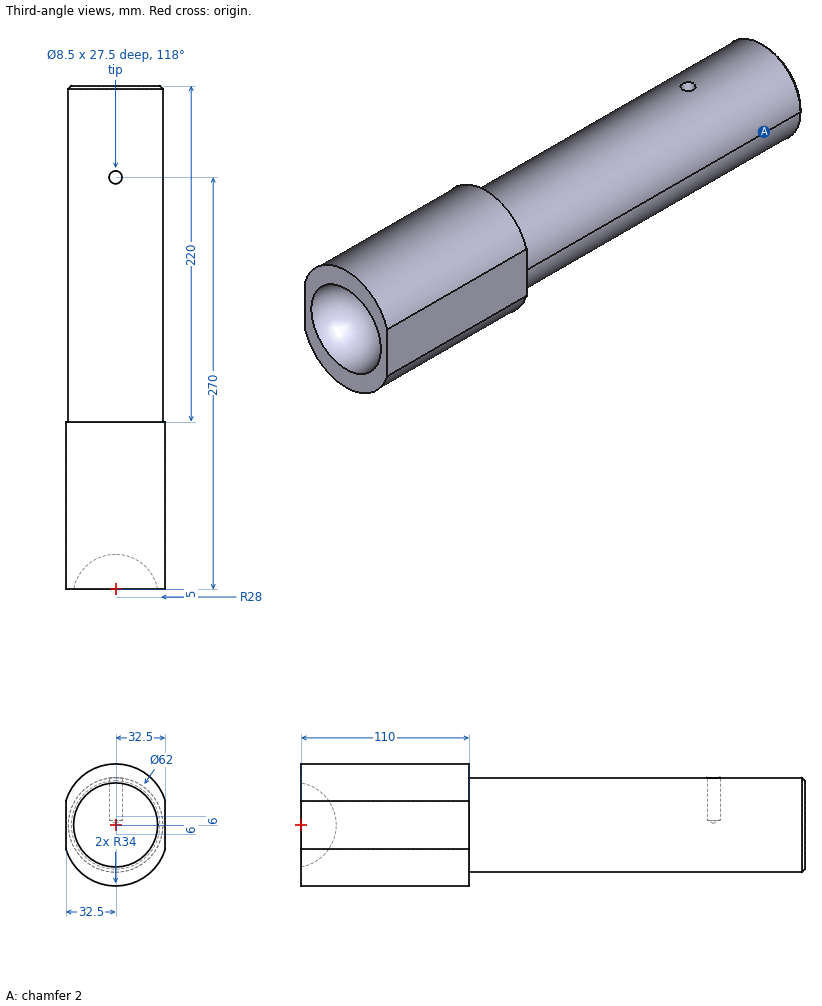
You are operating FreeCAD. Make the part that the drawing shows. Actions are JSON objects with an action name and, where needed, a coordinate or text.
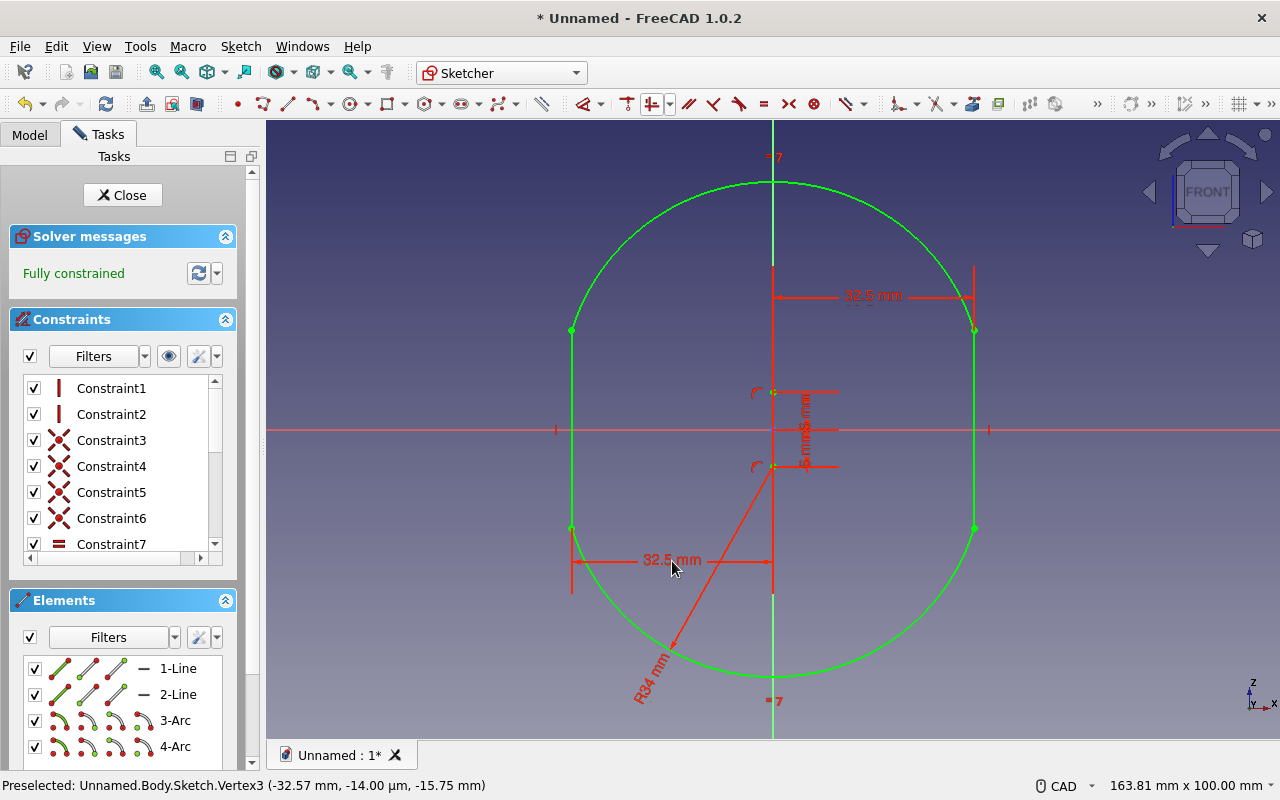
{"action": "left_click", "coordinate": [123, 195]}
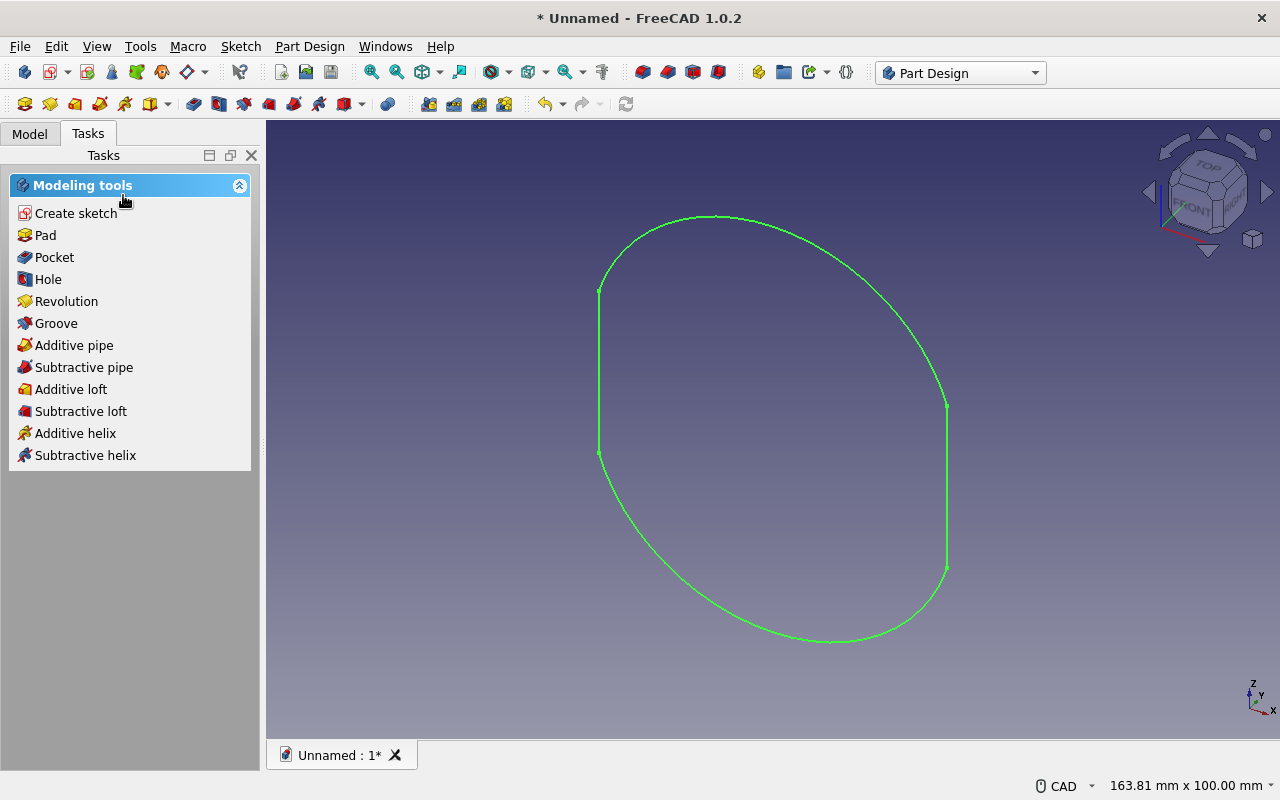
{"action": "left_click", "coordinate": [25, 104]}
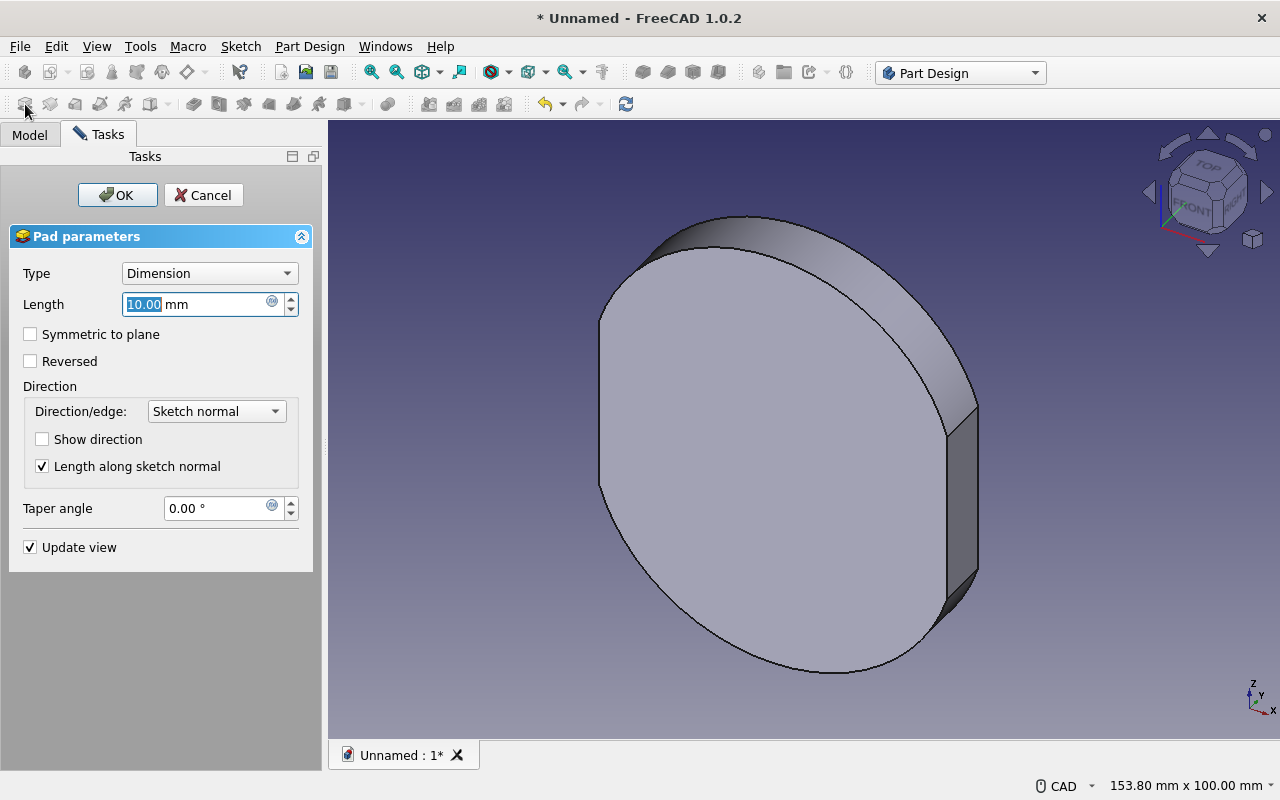
{"action": "type", "text": "110"}
{"action": "key", "text": "Tab"}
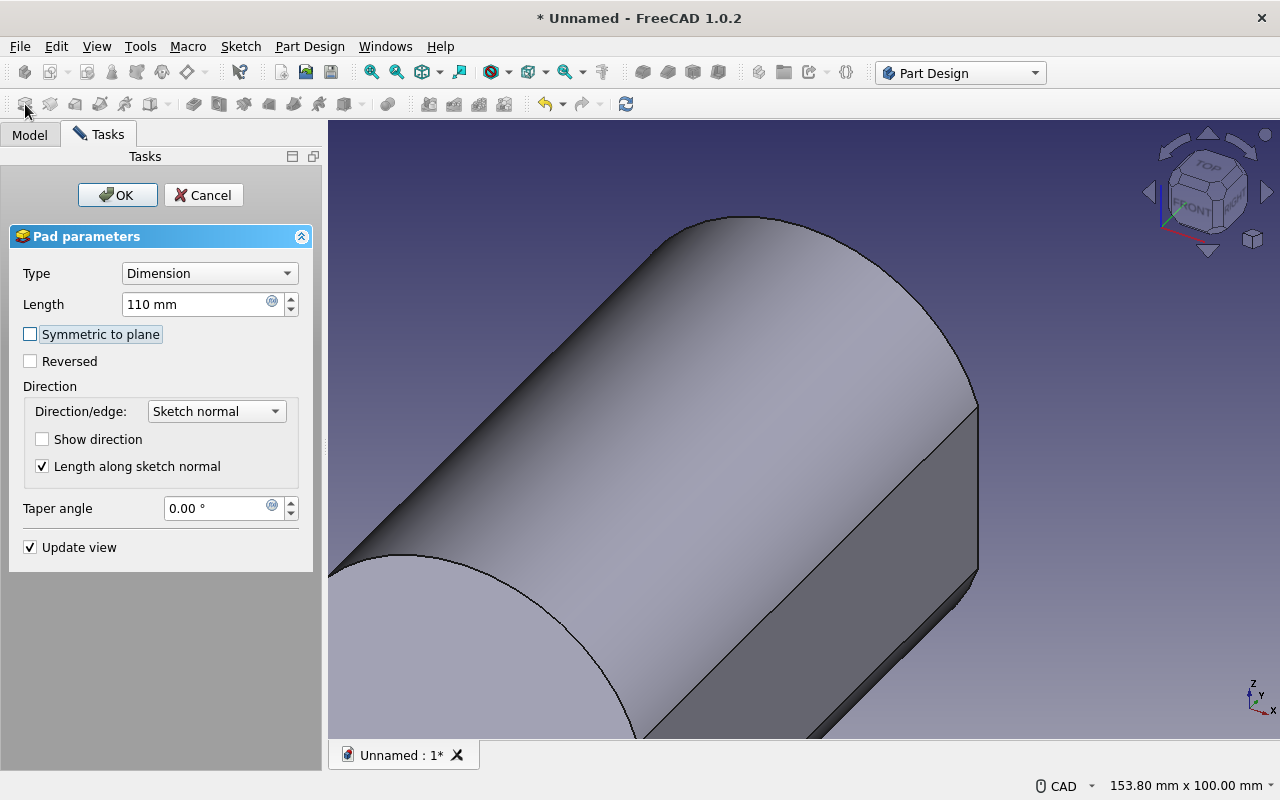
{"action": "left_click", "coordinate": [31, 361]}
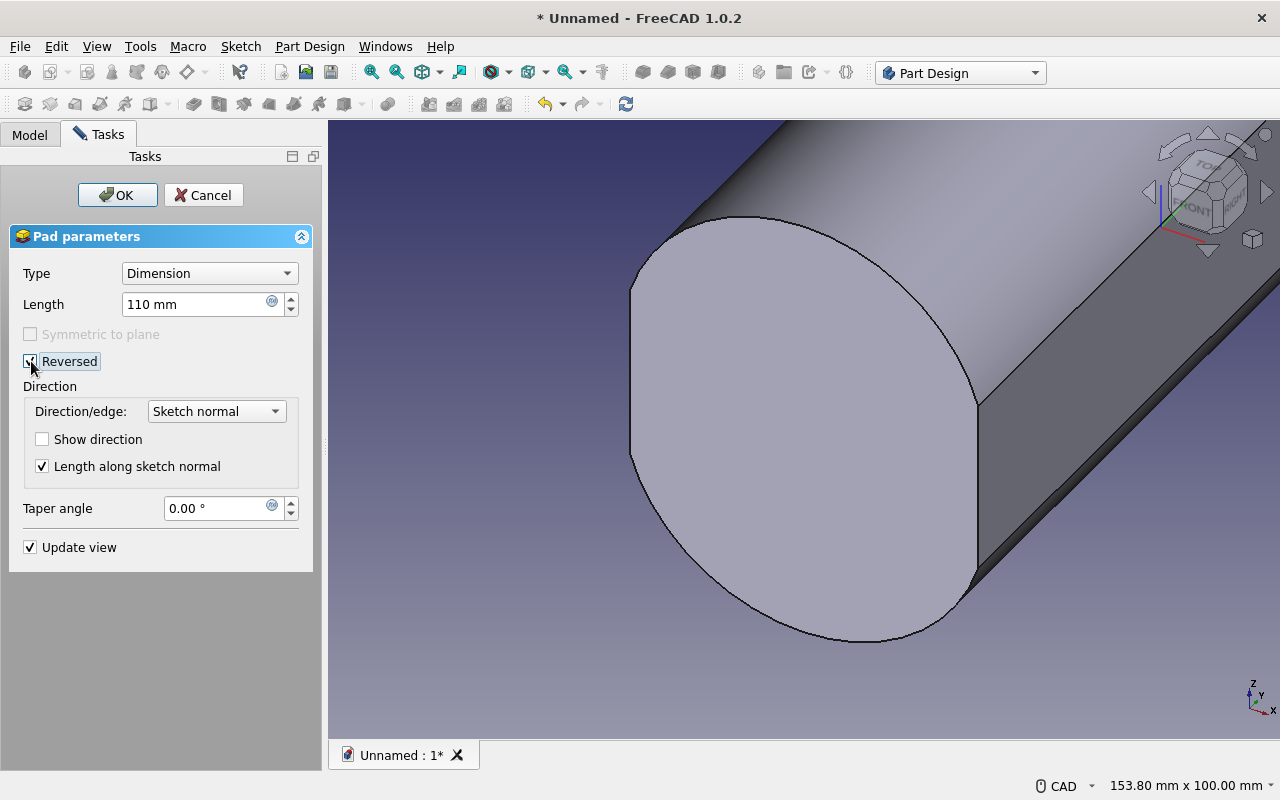
{"action": "left_click", "coordinate": [118, 195]}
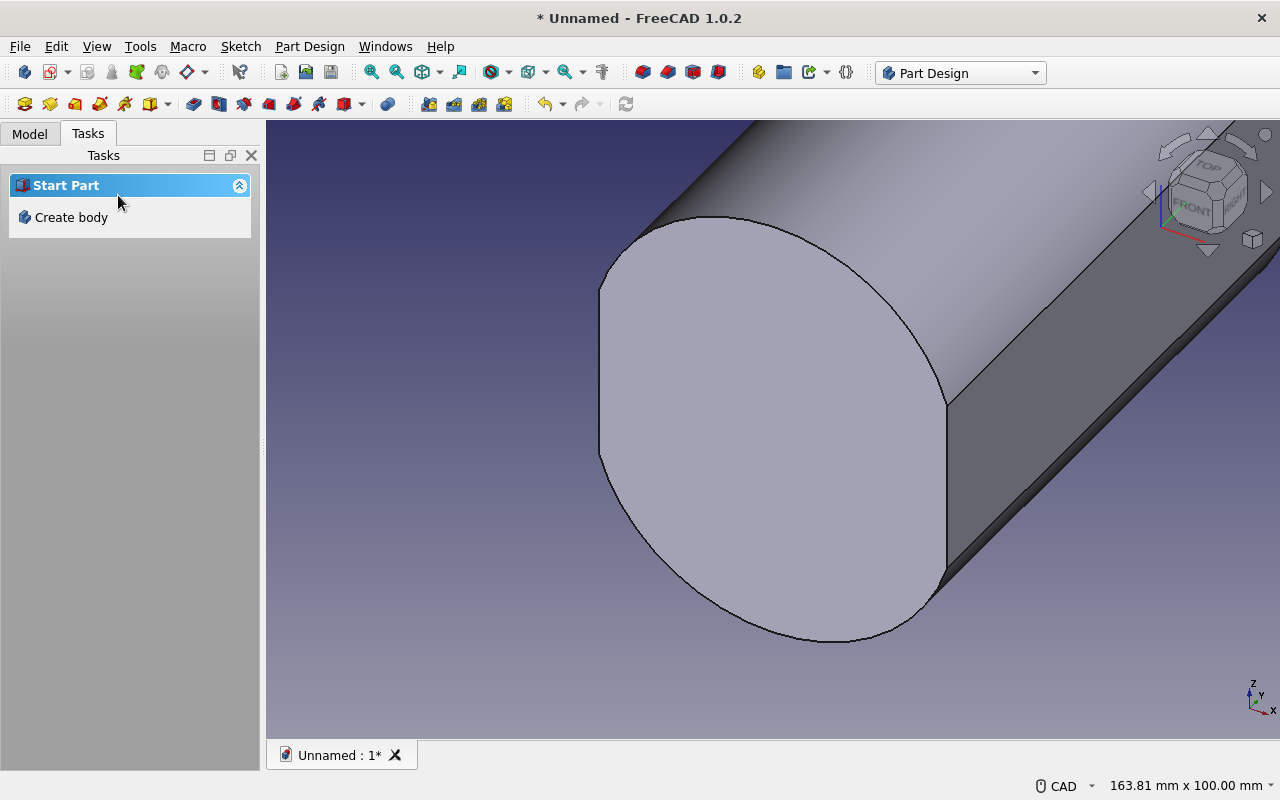
{"action": "left_click", "coordinate": [372, 72]}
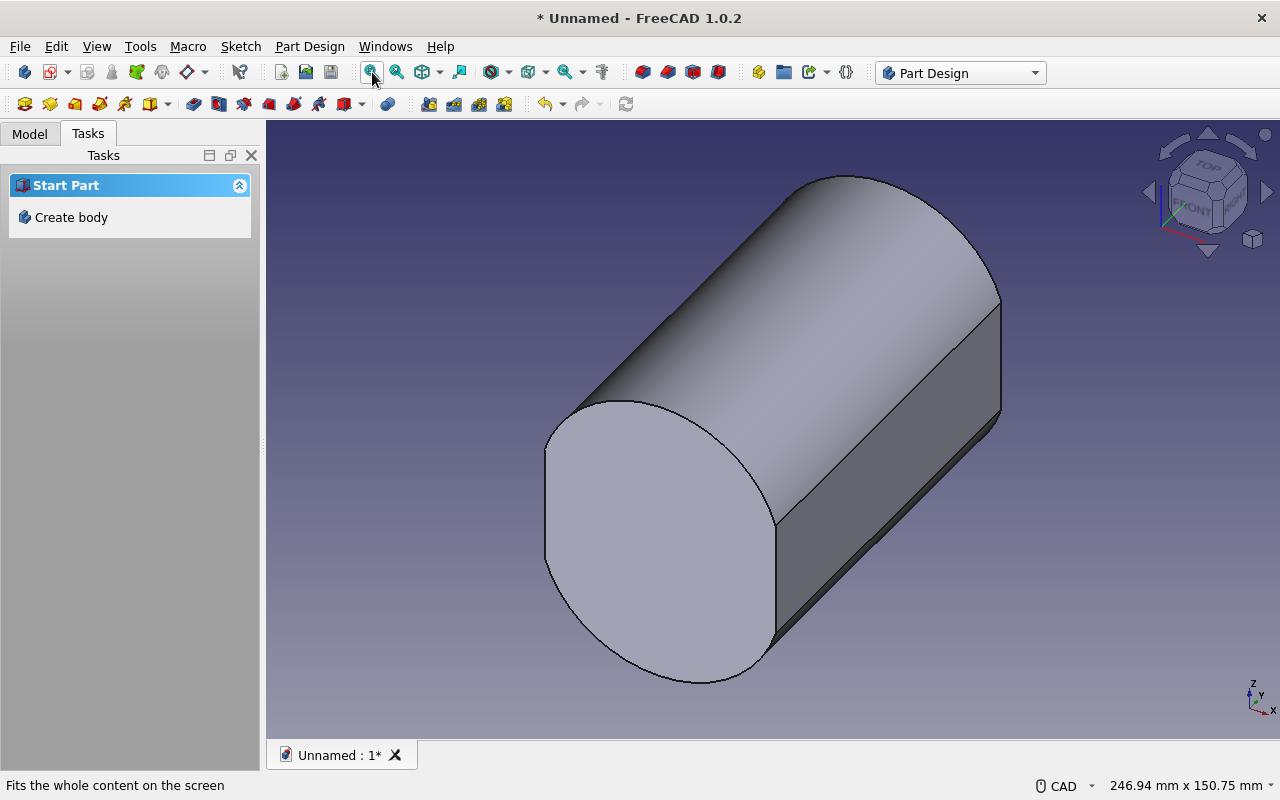
{"action": "key", "text": "4"}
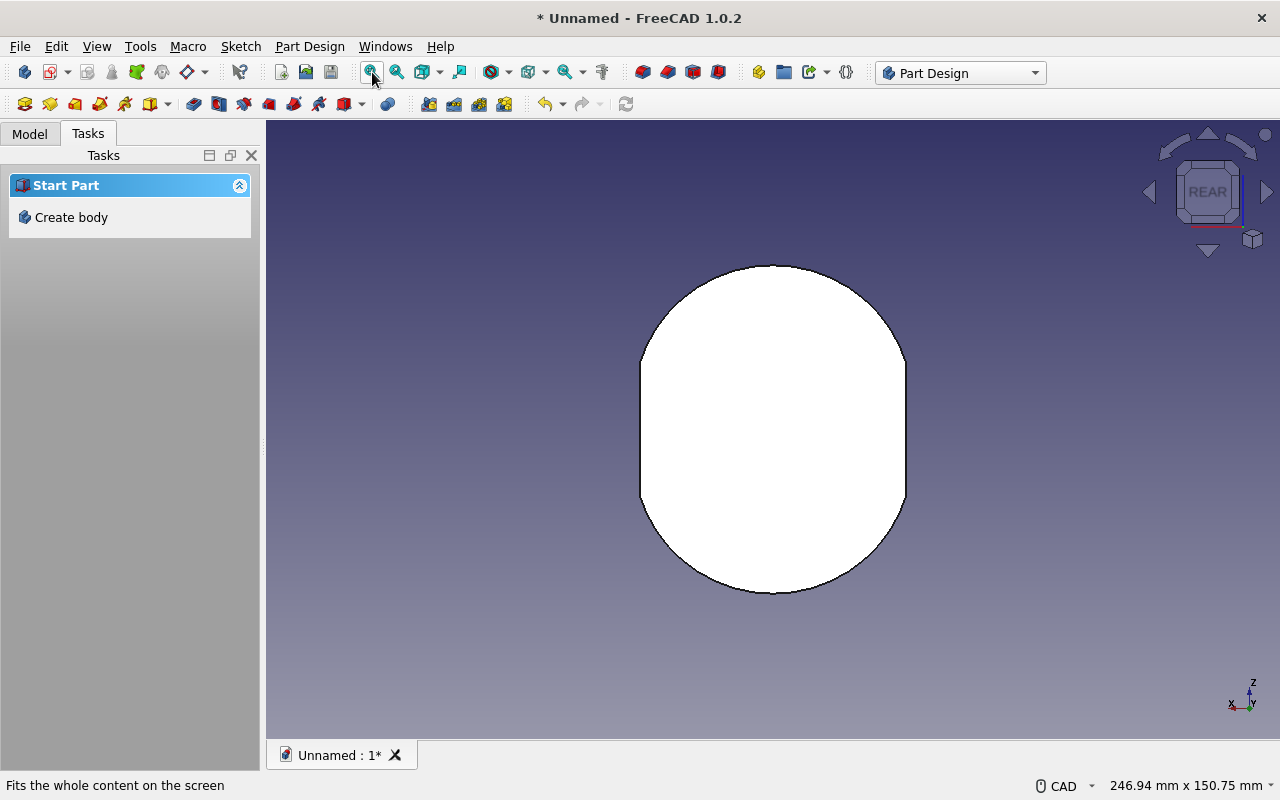
{"action": "left_click", "coordinate": [773, 429]}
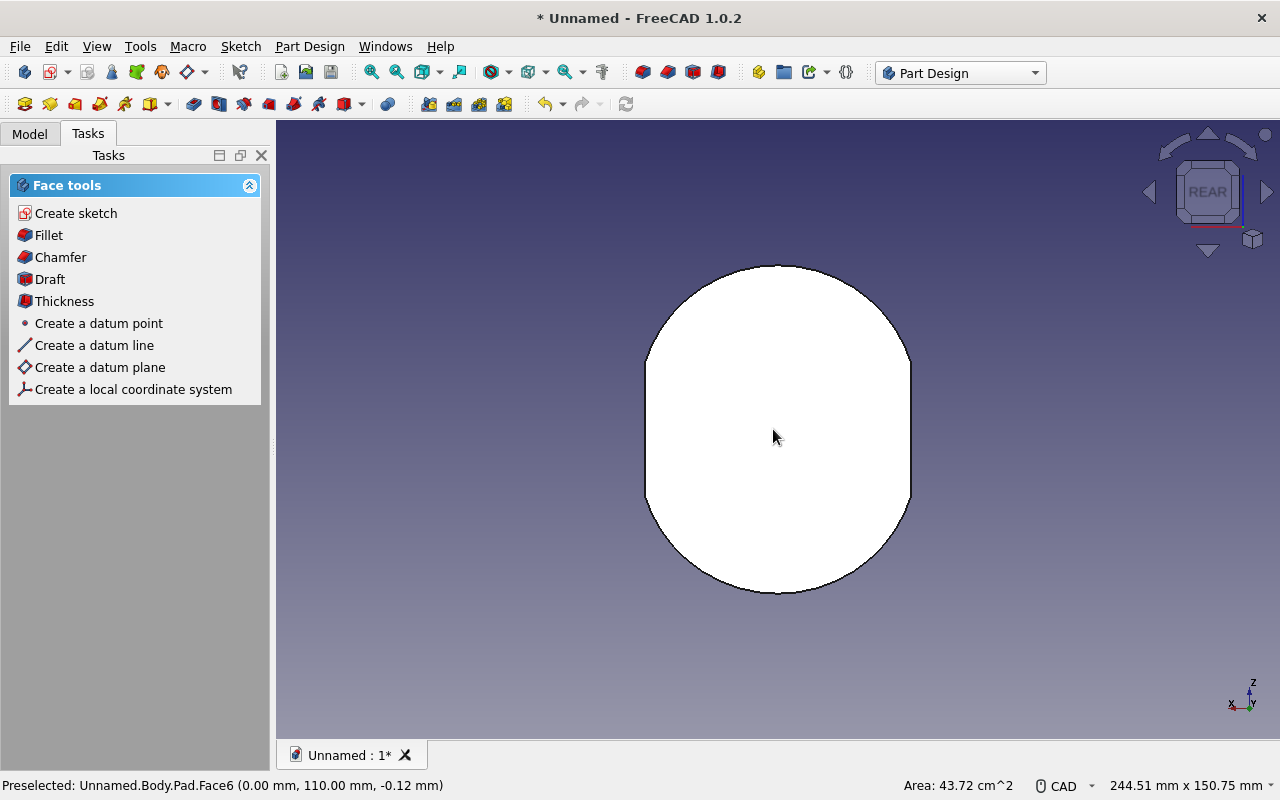
{"action": "left_click", "coordinate": [50, 72]}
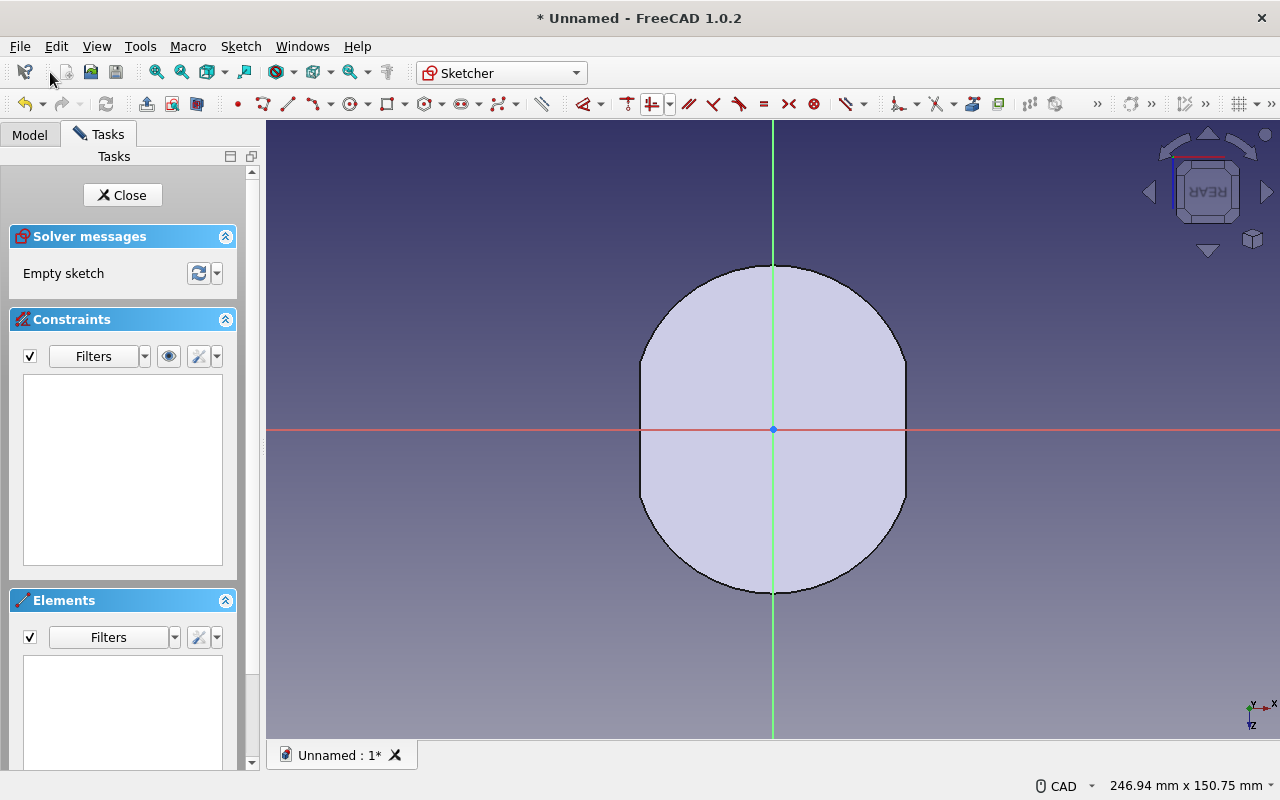
{"action": "scroll", "coordinate": [912, 429], "scroll_direction": "up", "scroll_amount": 2}